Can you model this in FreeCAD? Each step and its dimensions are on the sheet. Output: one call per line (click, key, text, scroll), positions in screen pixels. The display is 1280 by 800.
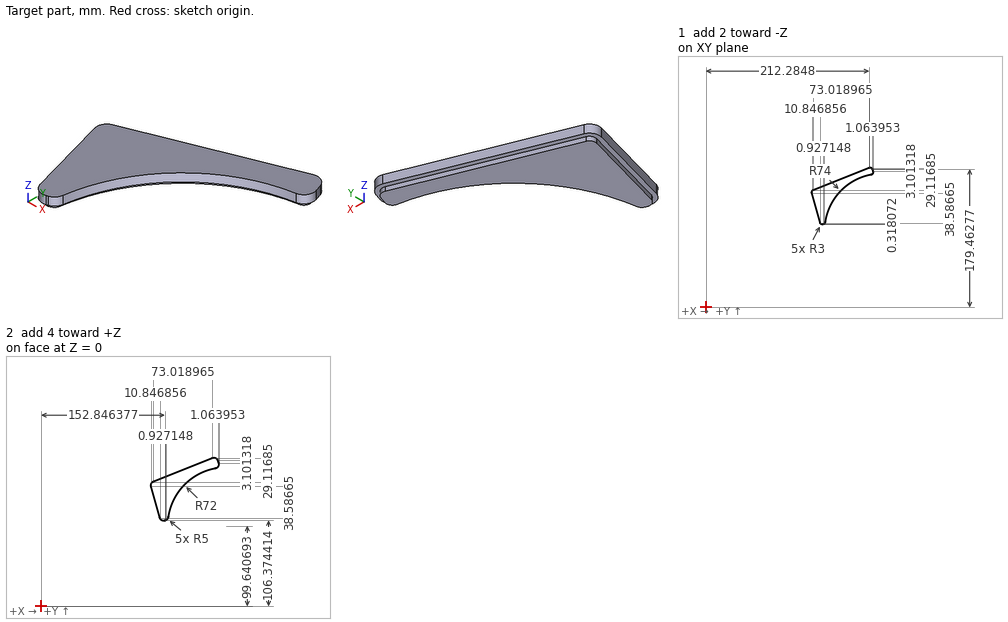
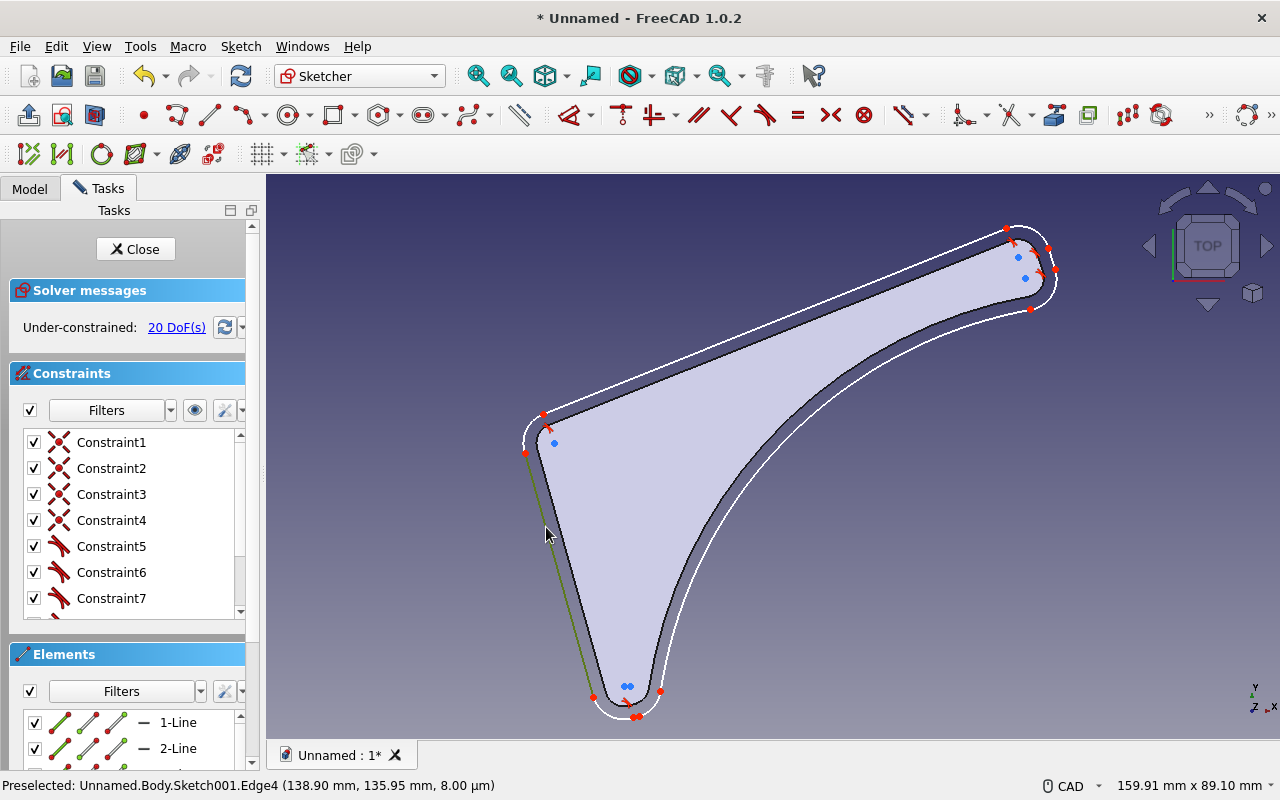
click(532, 422)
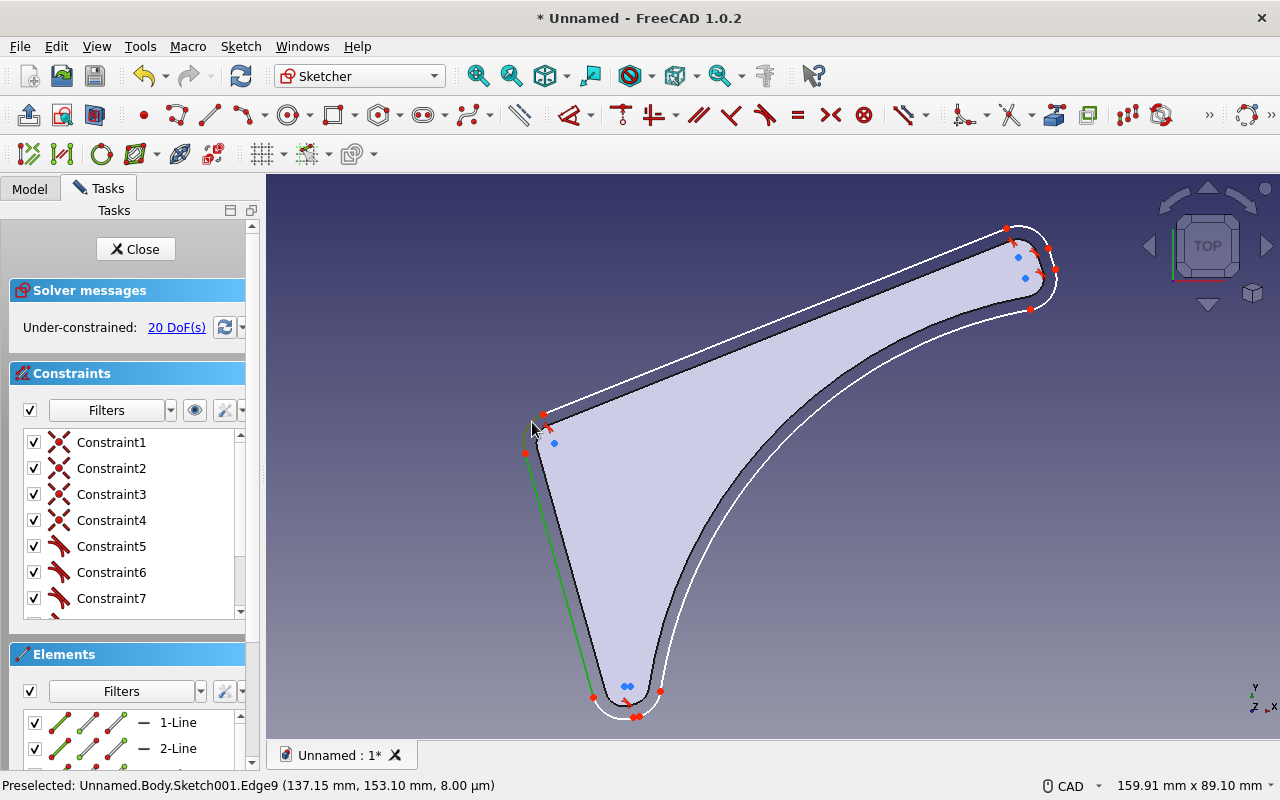
click(765, 116)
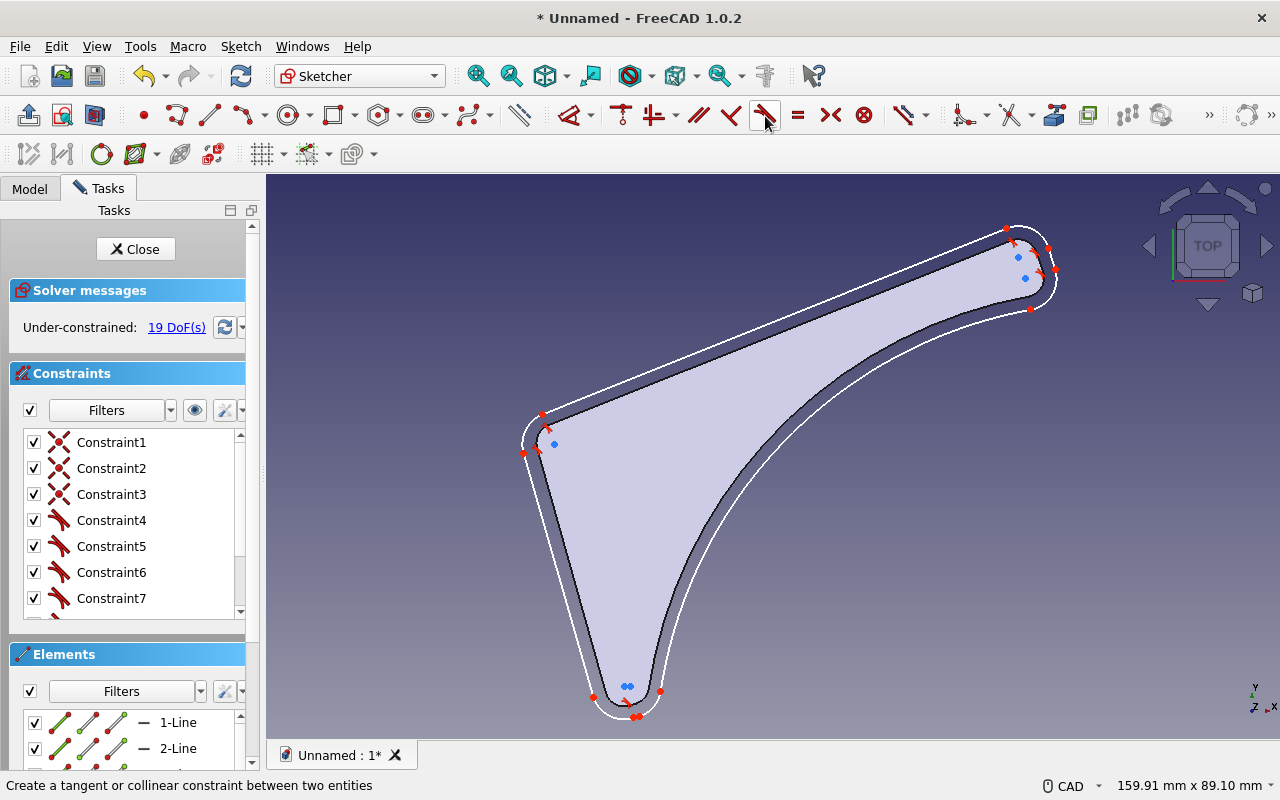
click(545, 527)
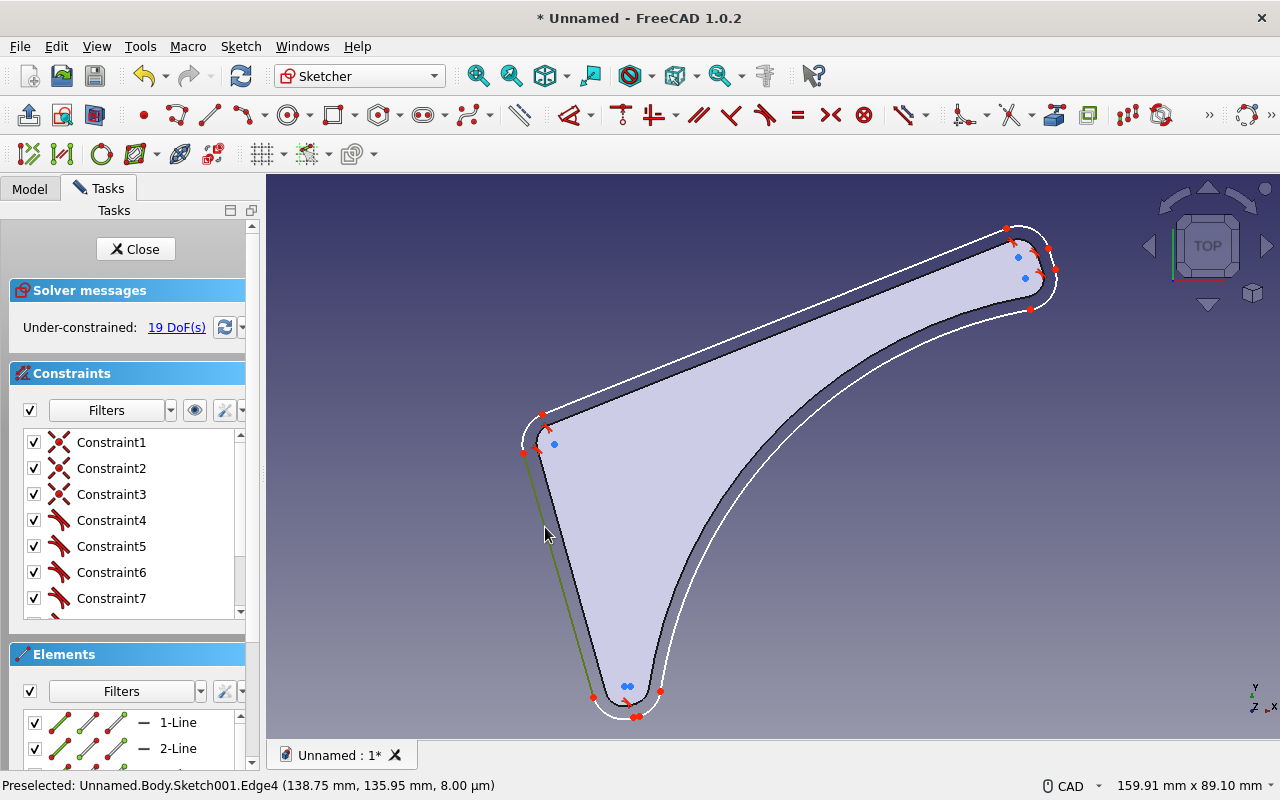
click(602, 710)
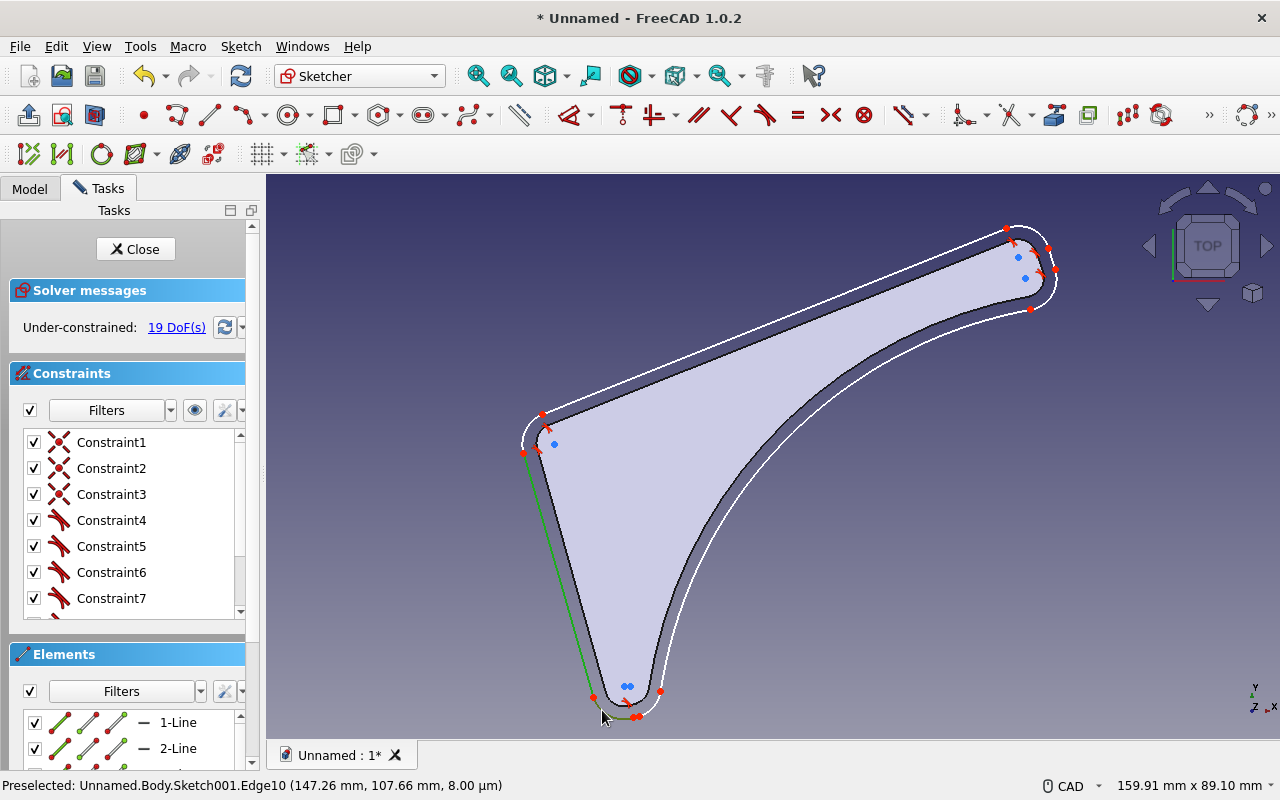
click(765, 116)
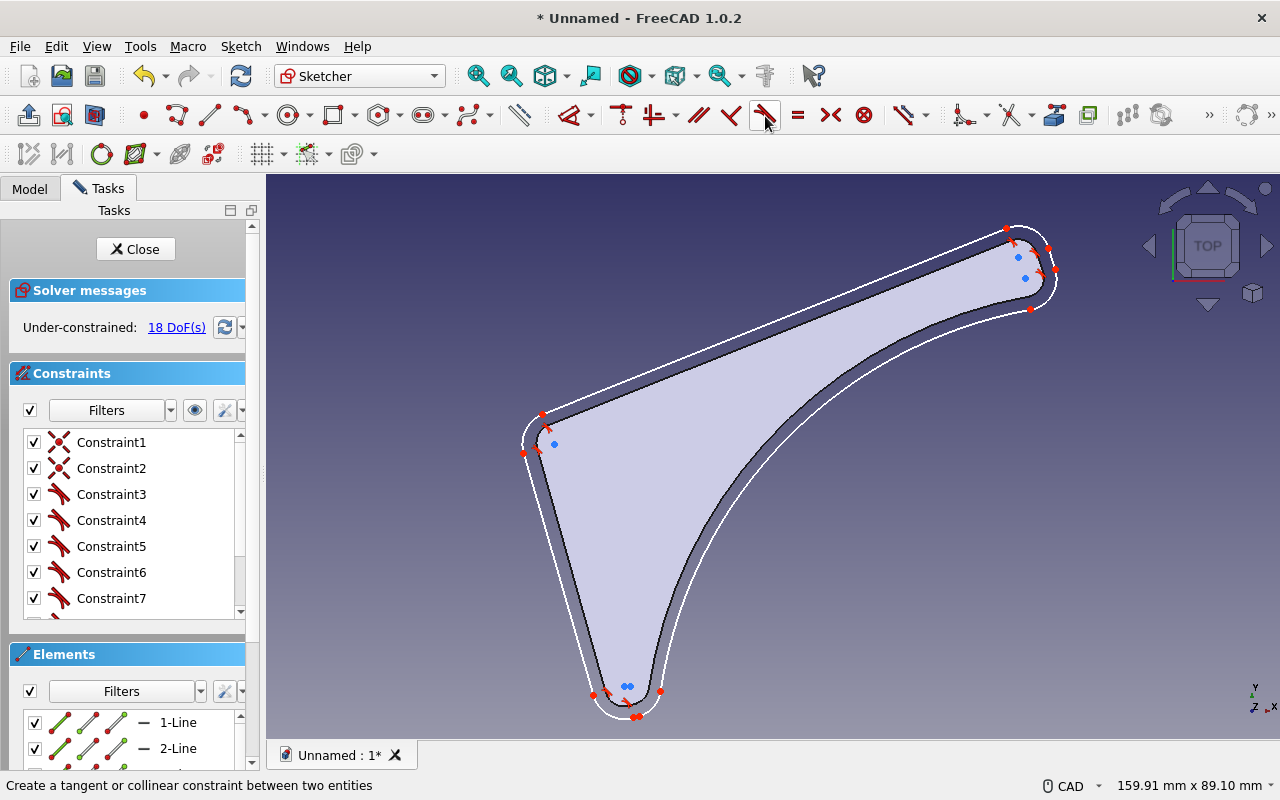
scroll(657, 702, up, 2)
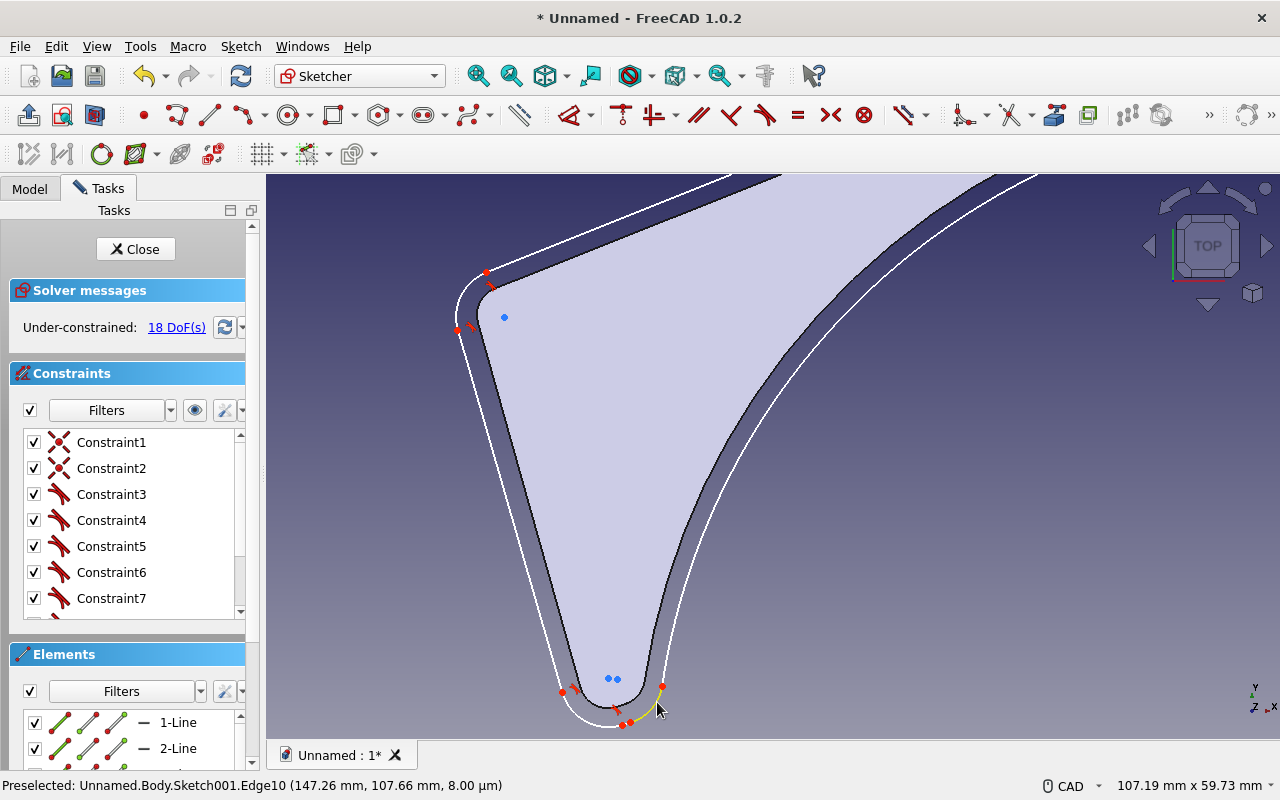
click(657, 701)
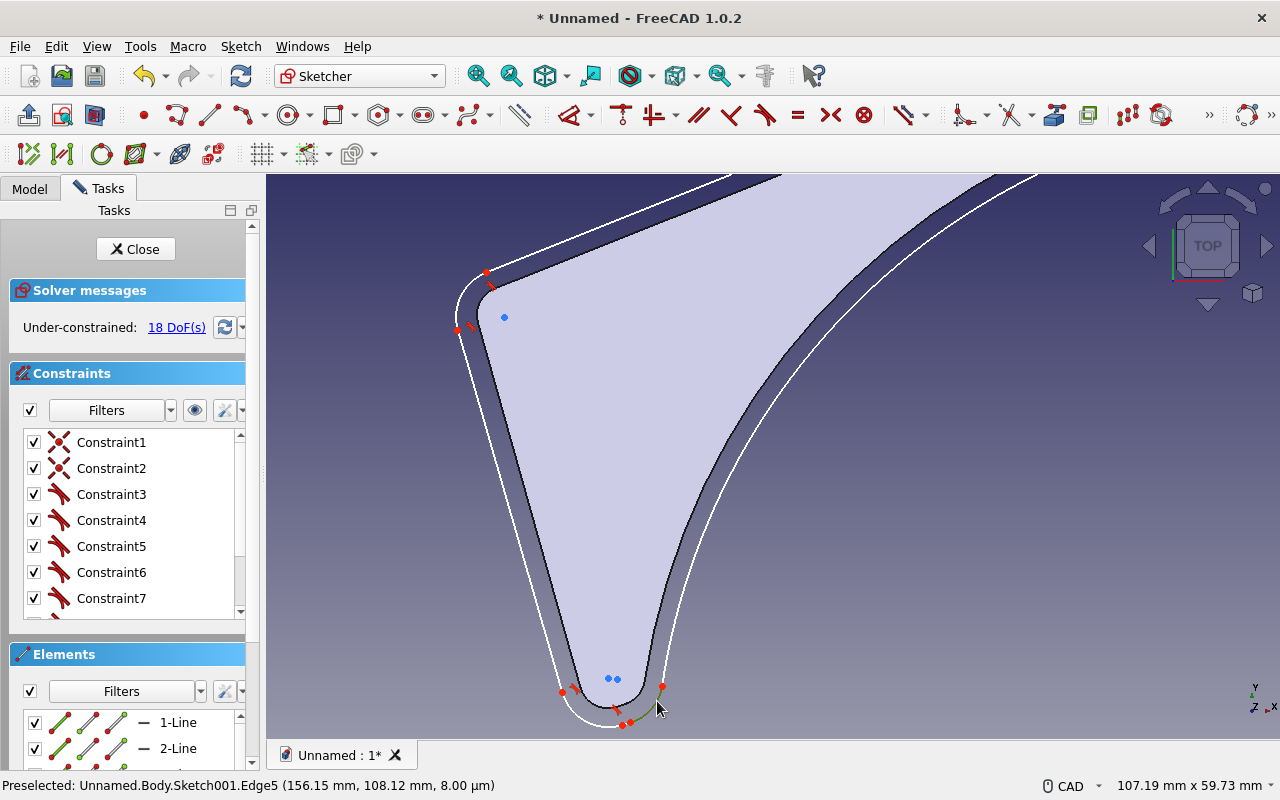
click(978, 207)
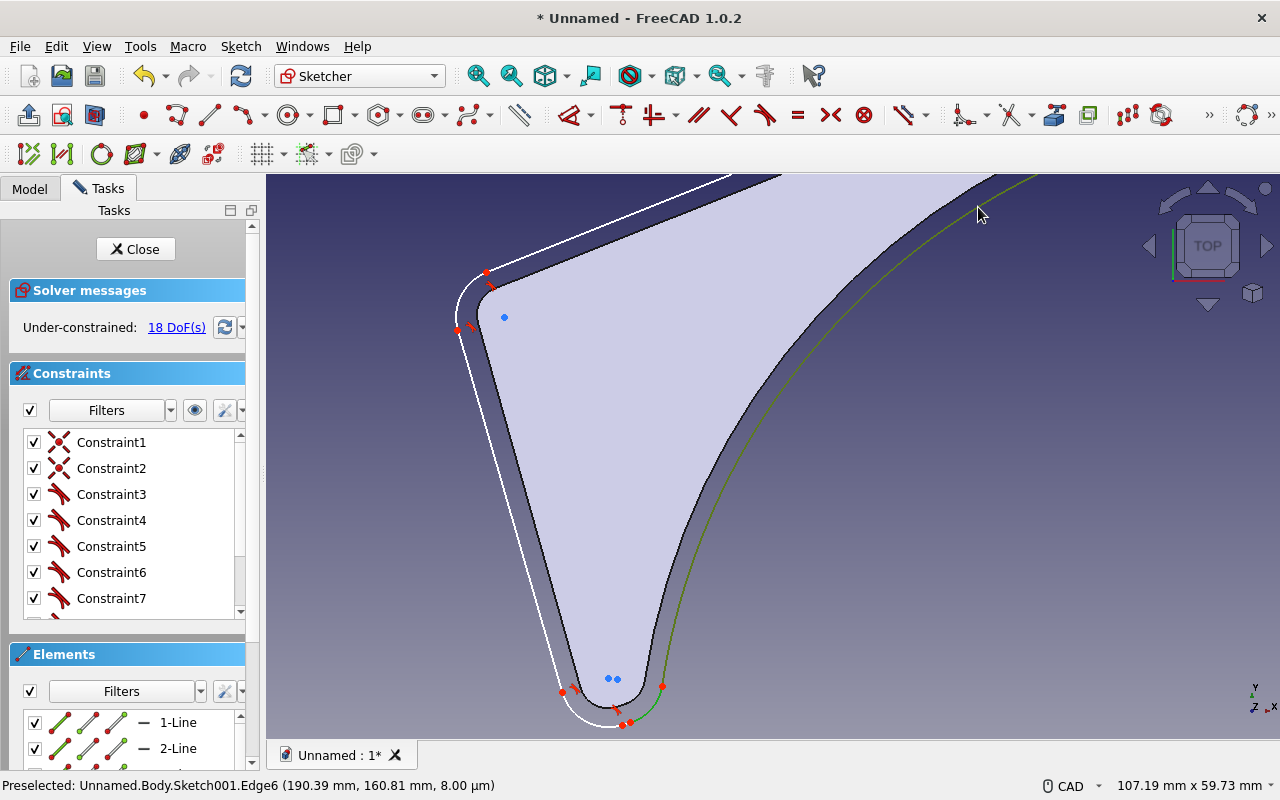
click(765, 116)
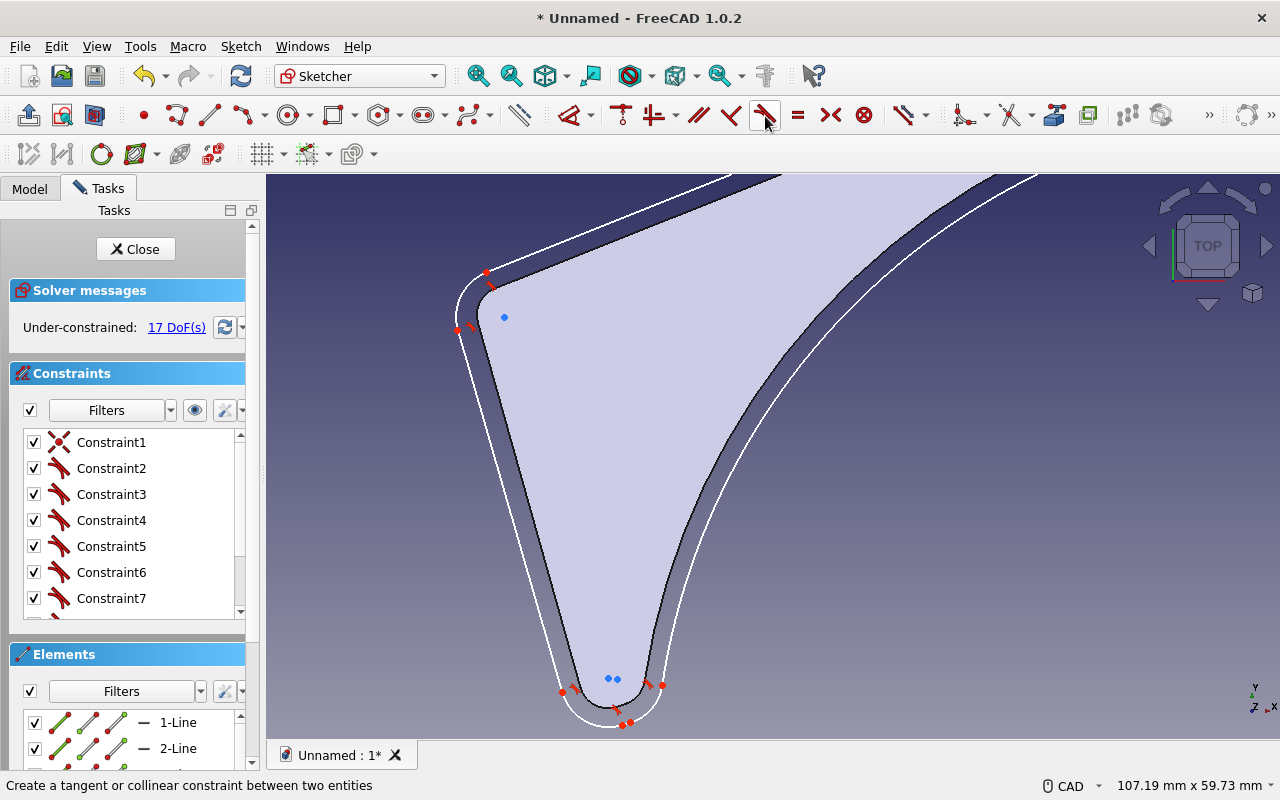
click(979, 207)